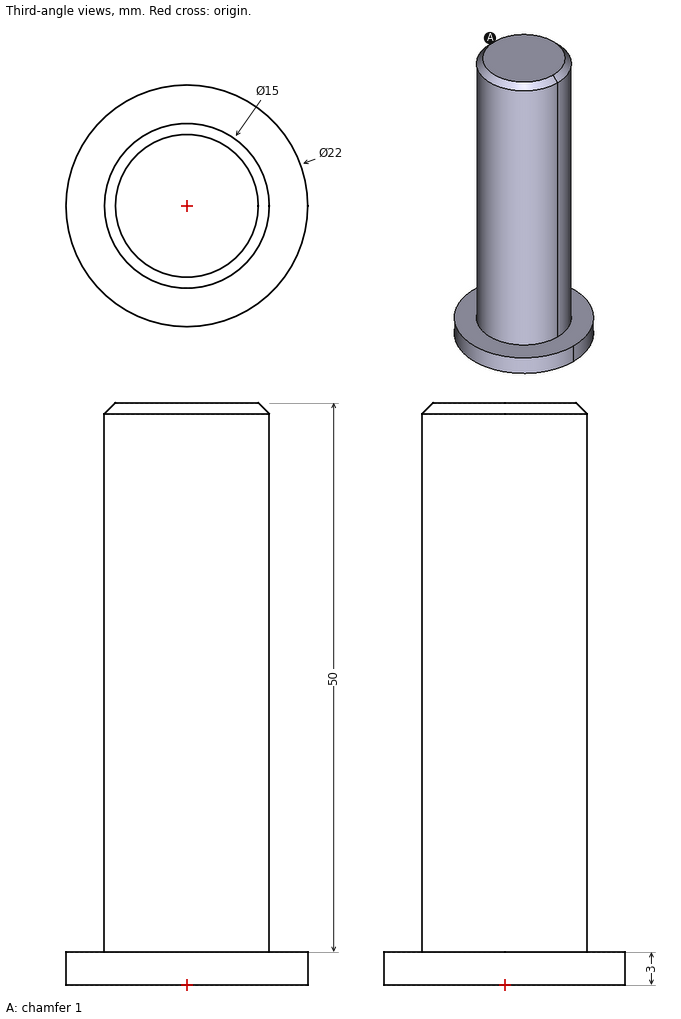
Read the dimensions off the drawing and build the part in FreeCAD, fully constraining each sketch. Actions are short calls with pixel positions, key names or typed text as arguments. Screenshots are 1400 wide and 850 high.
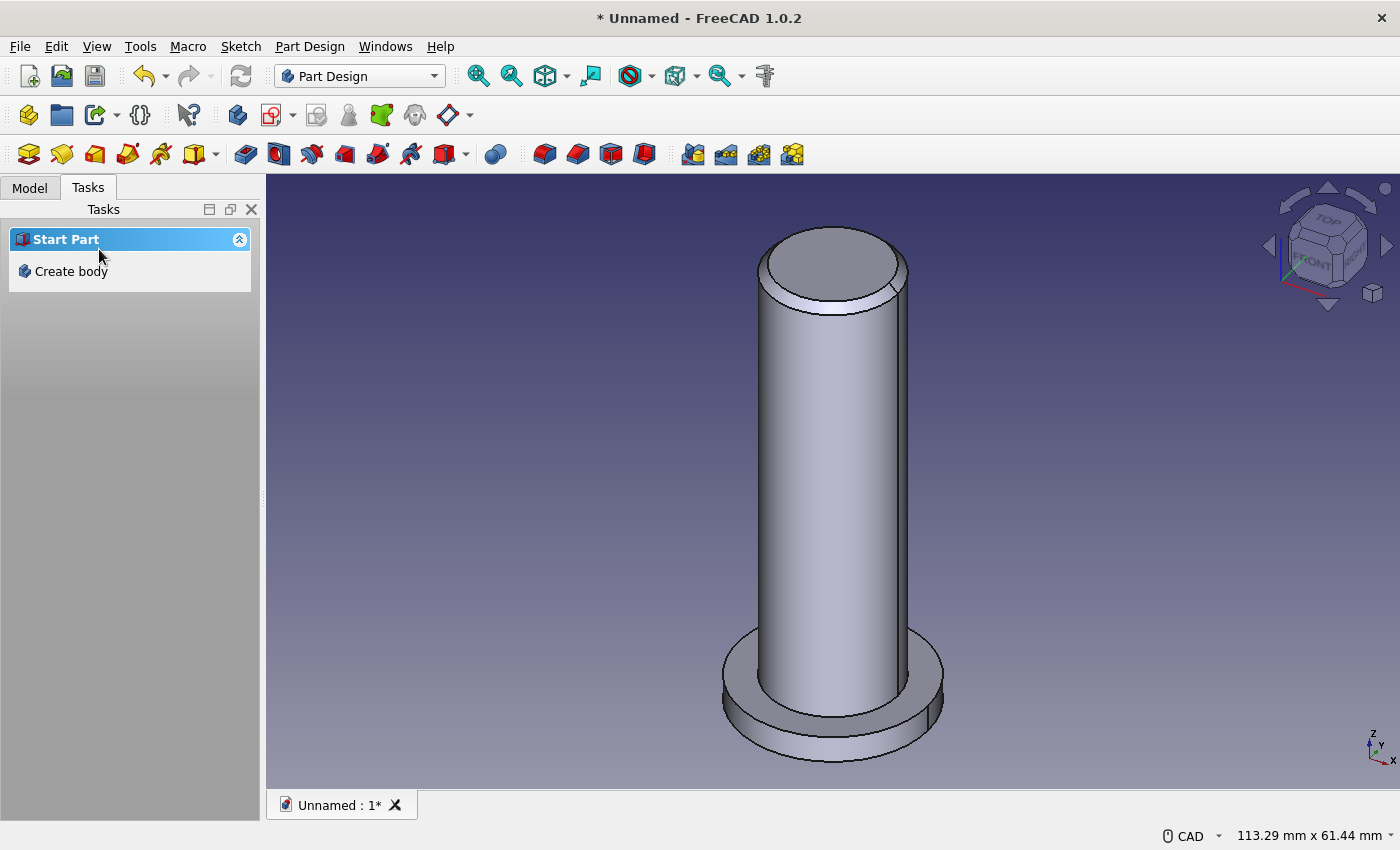
key(0)